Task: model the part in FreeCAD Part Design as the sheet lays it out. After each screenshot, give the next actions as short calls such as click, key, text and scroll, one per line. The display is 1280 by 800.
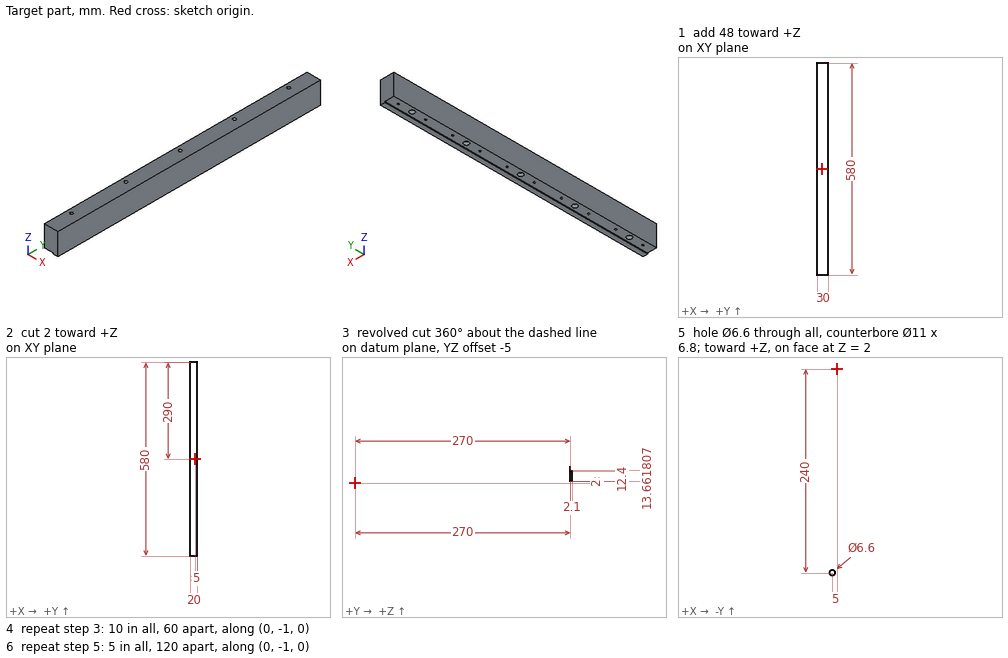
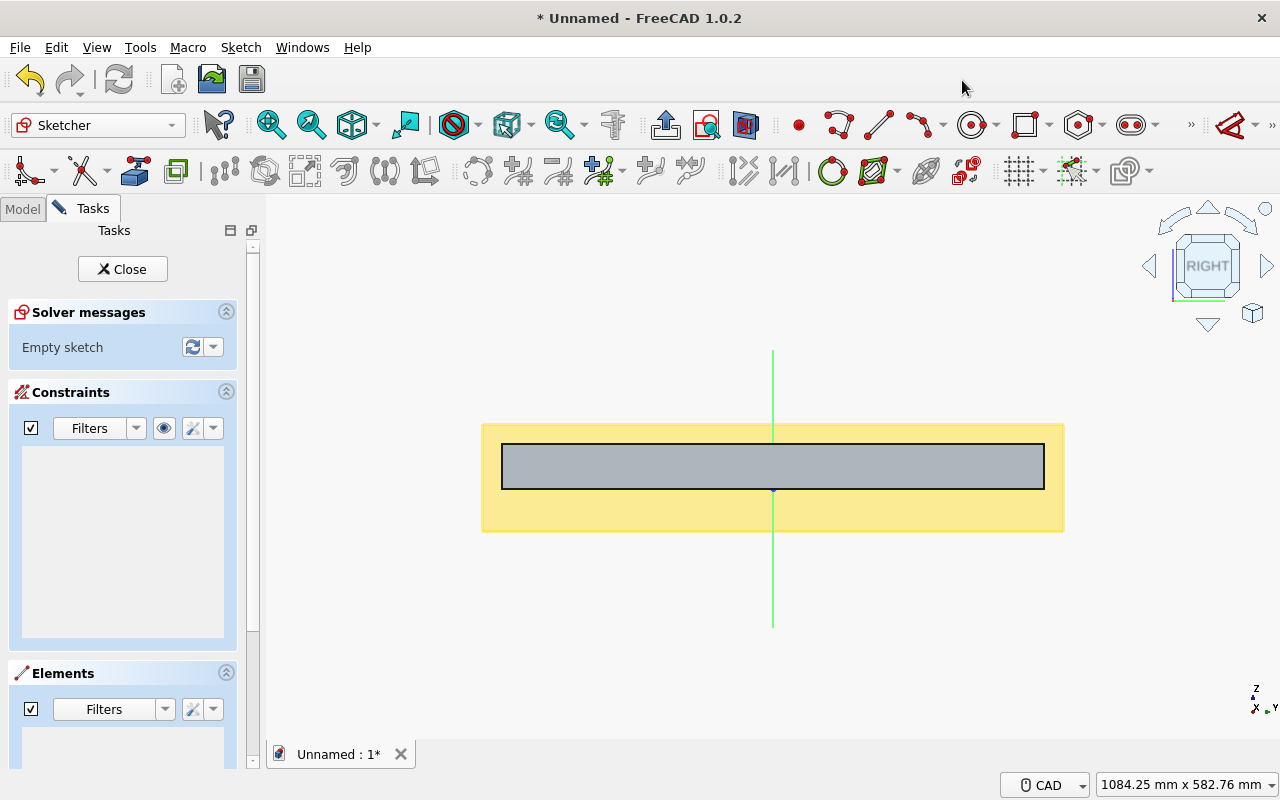
click(746, 126)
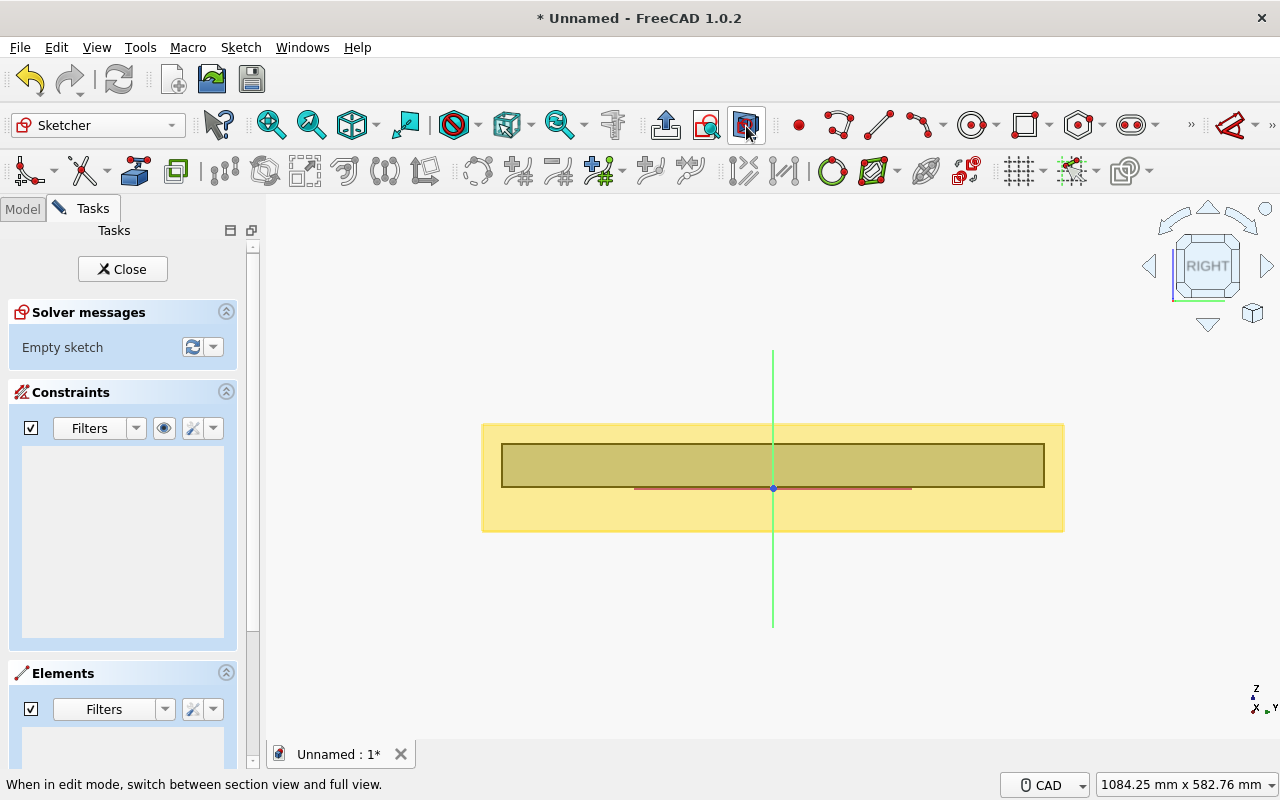
scroll(1043, 479, up, 15)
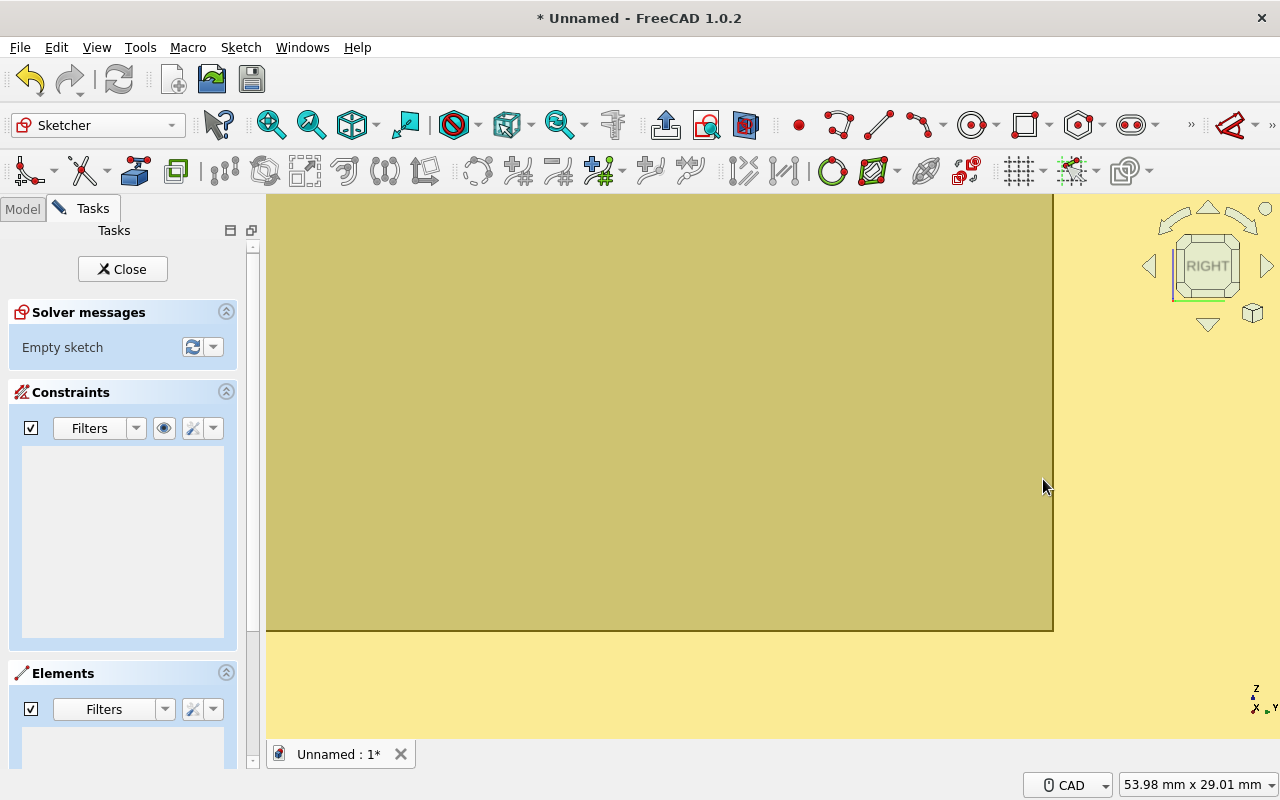
key(g)
key(m)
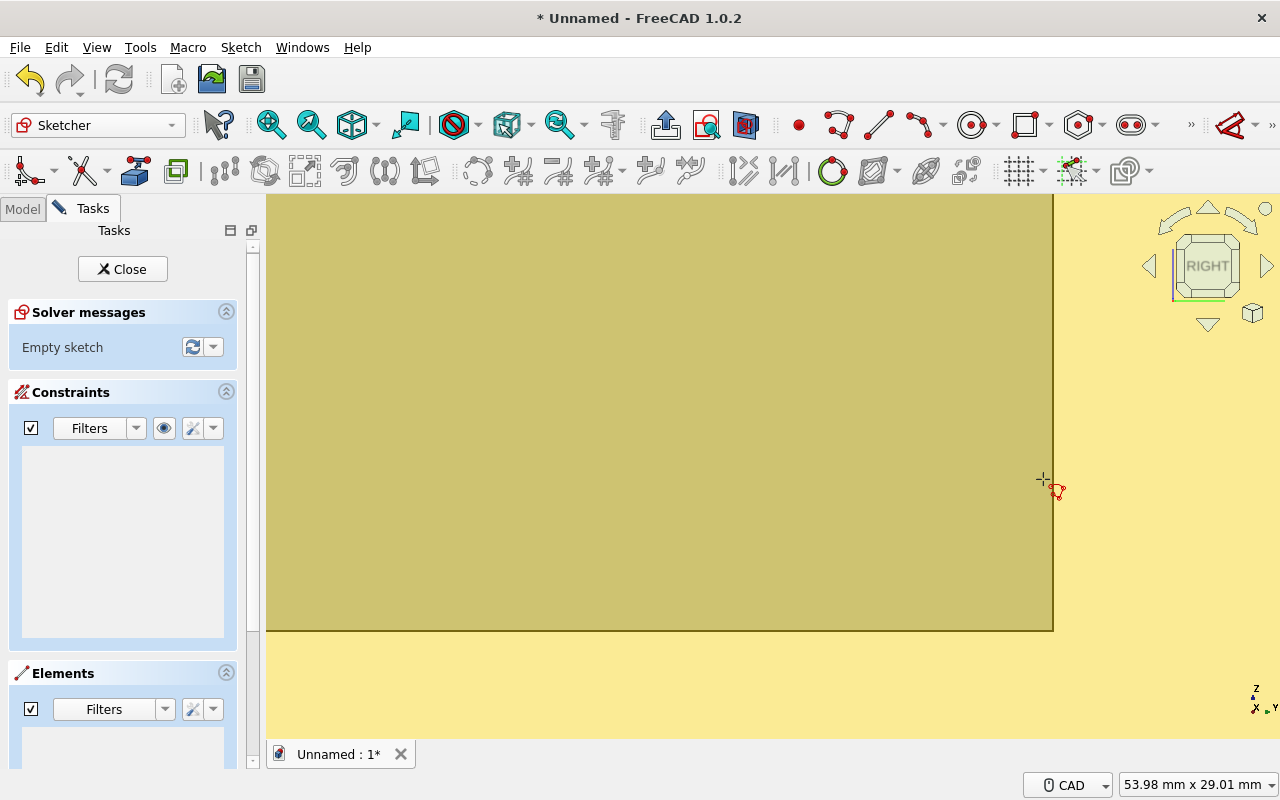
click(677, 631)
click(716, 631)
click(716, 398)
click(677, 375)
click(677, 632)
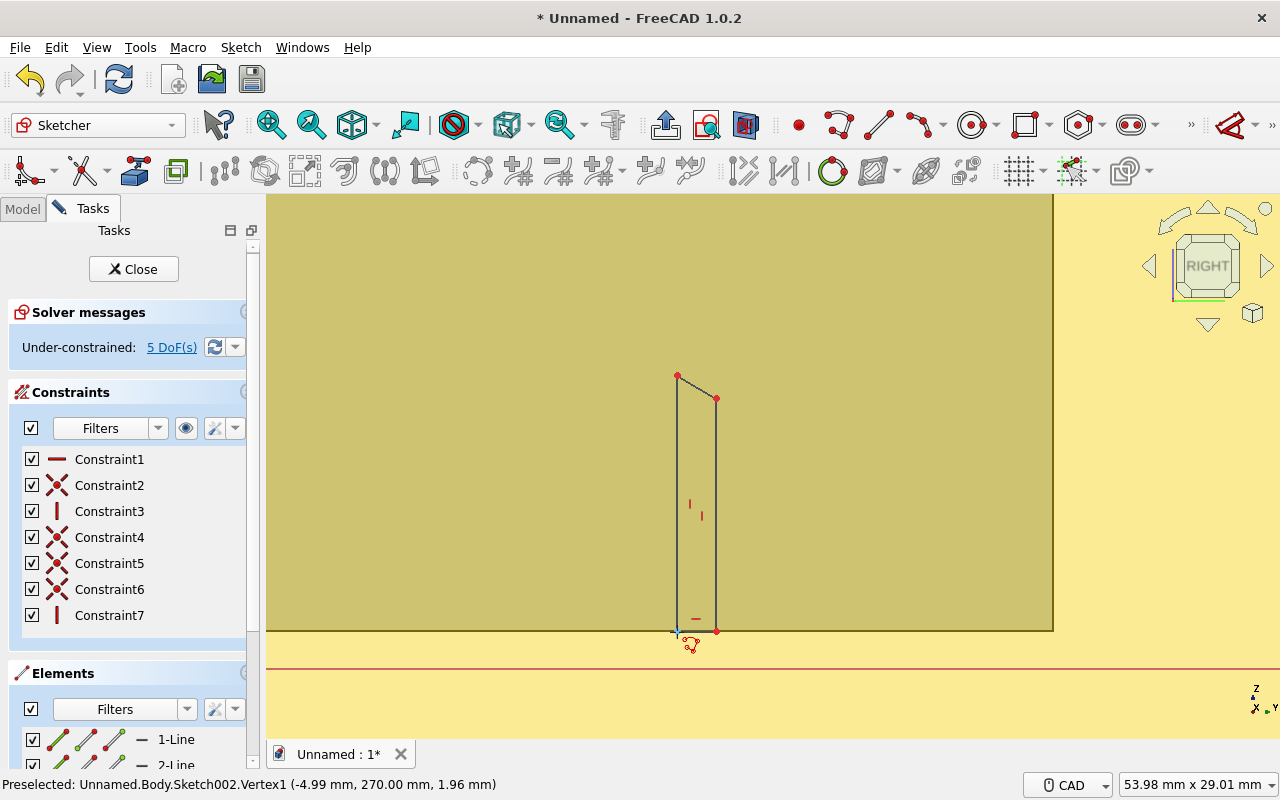
key(g)
key(l)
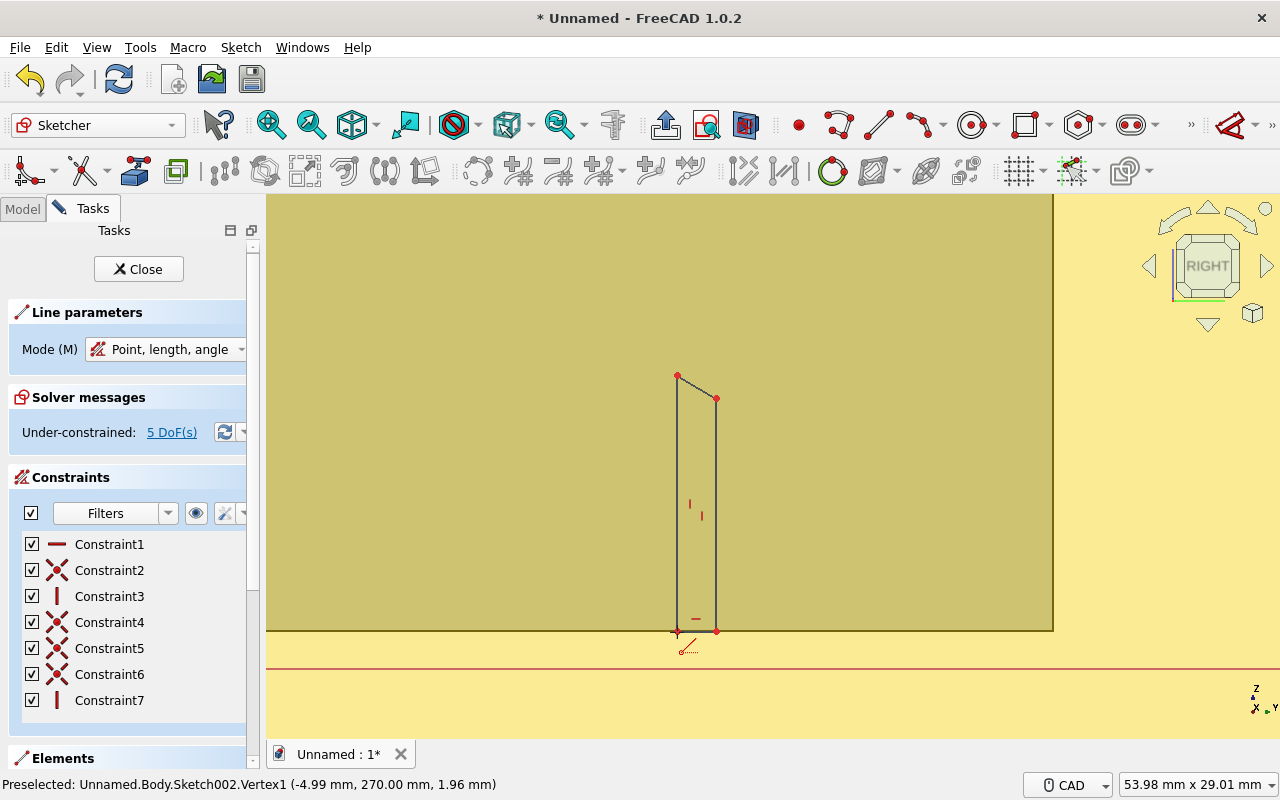
click(677, 349)
click(677, 272)
key(Escape)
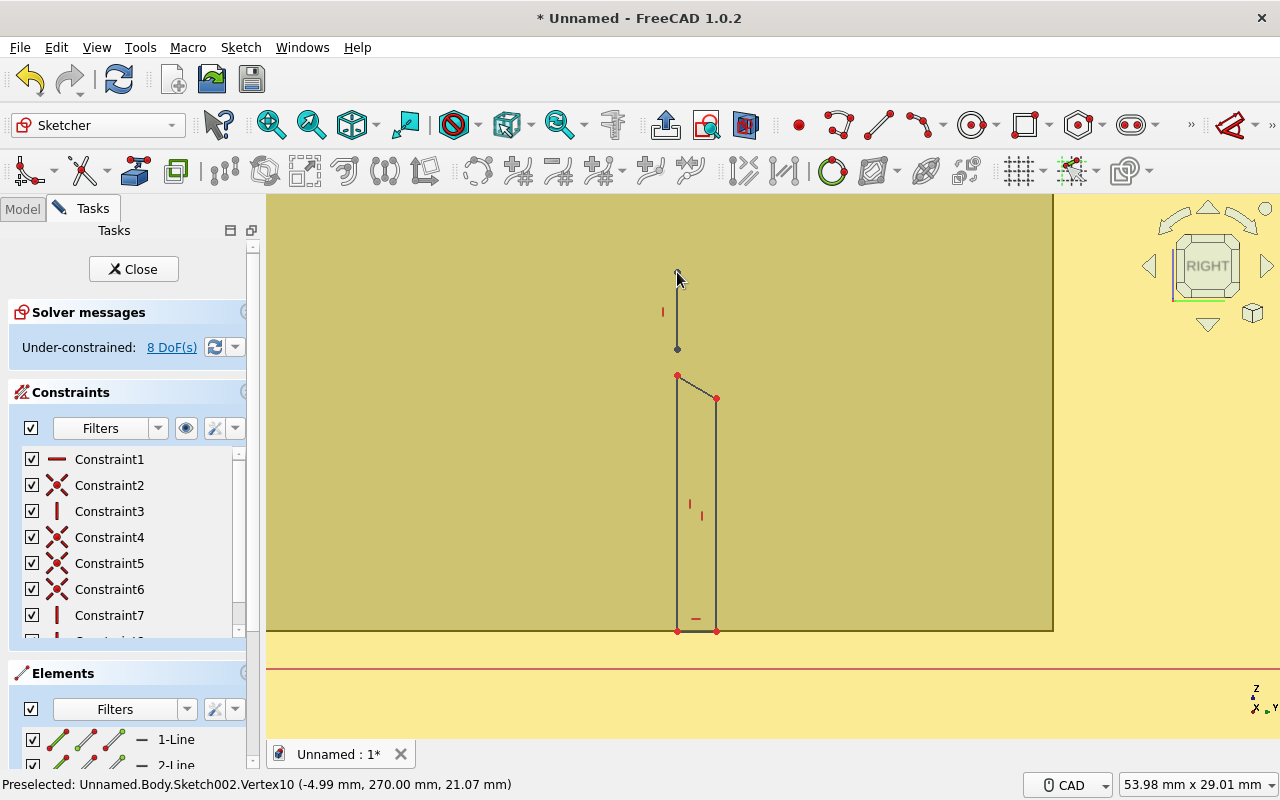
click(677, 327)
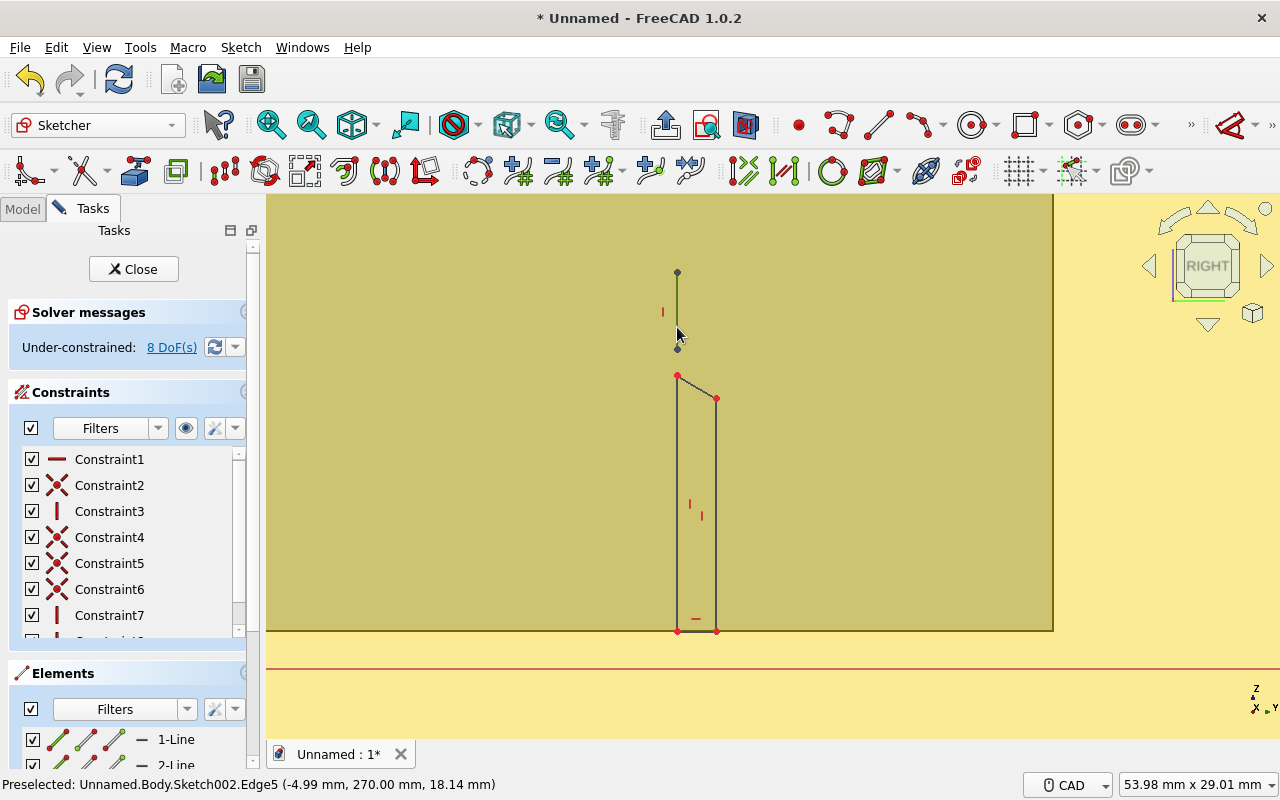
key(g)
key(n)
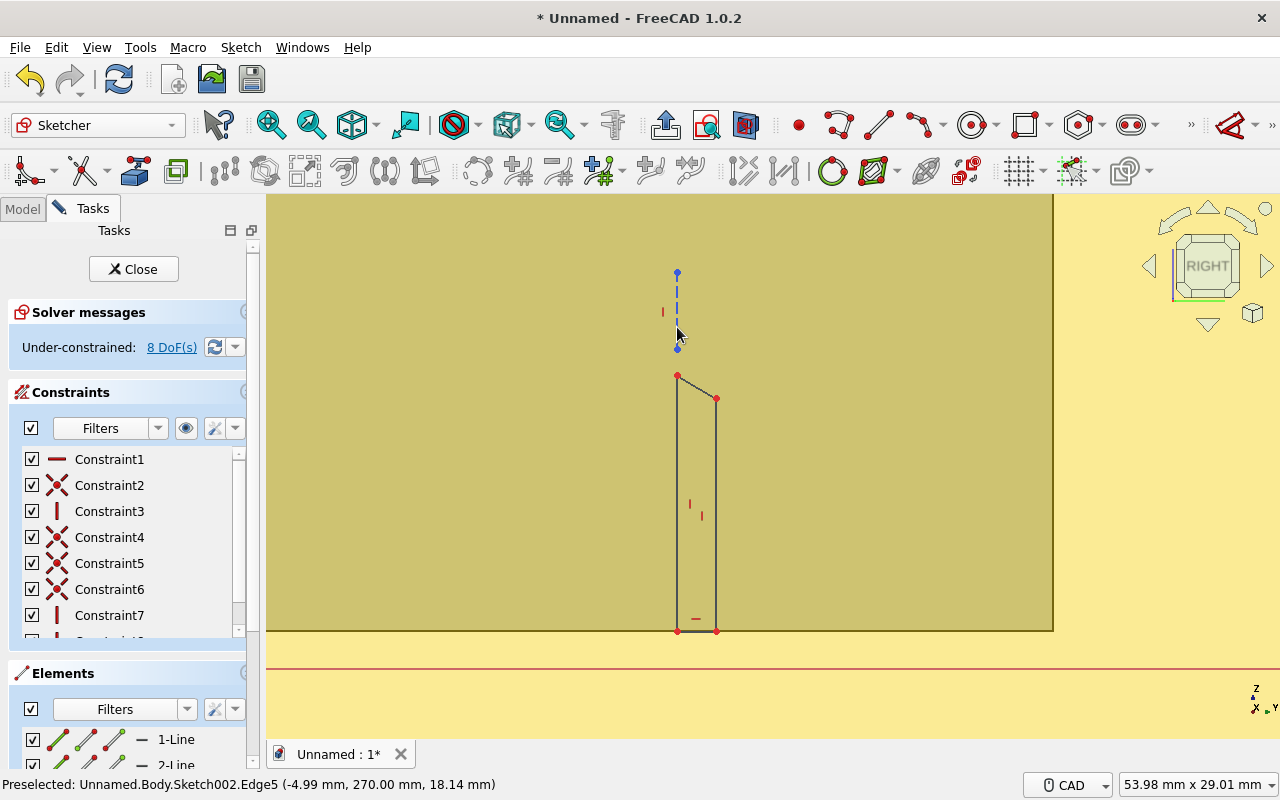
click(1230, 126)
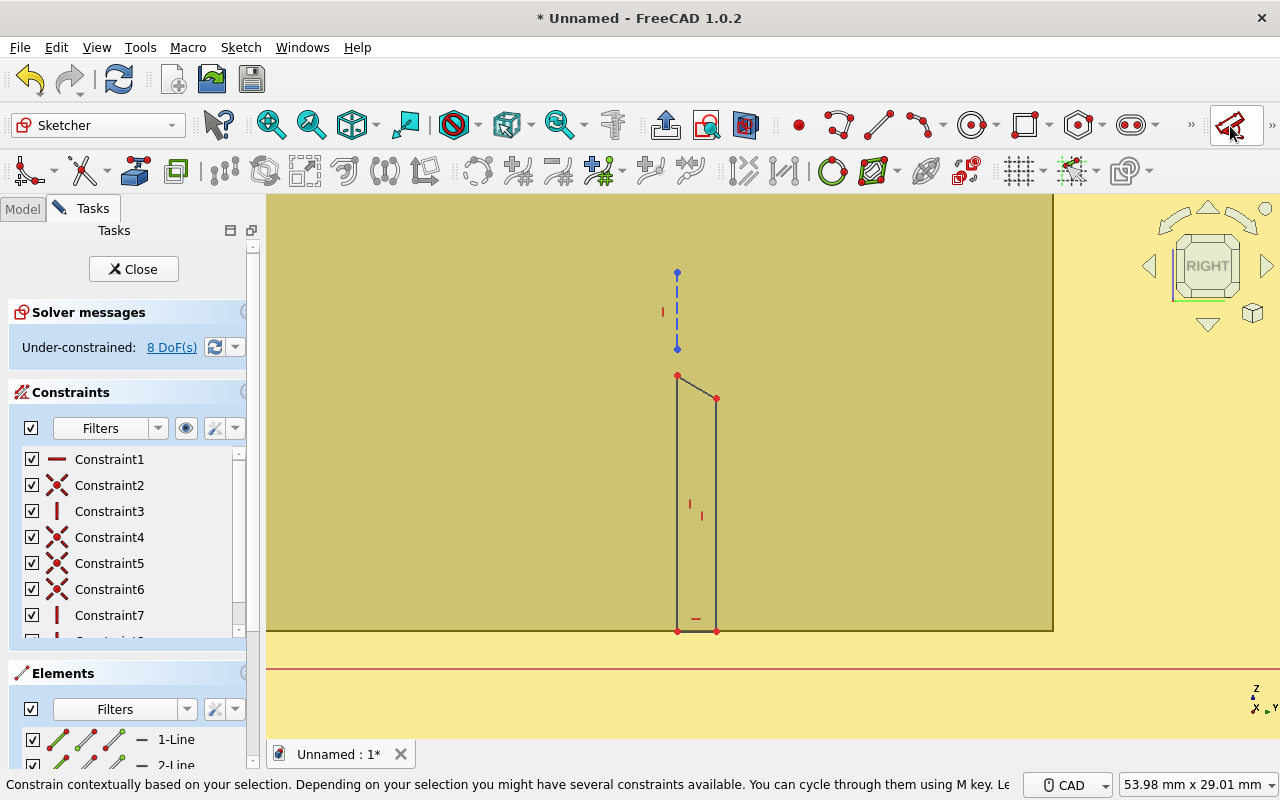
click(677, 632)
click(711, 650)